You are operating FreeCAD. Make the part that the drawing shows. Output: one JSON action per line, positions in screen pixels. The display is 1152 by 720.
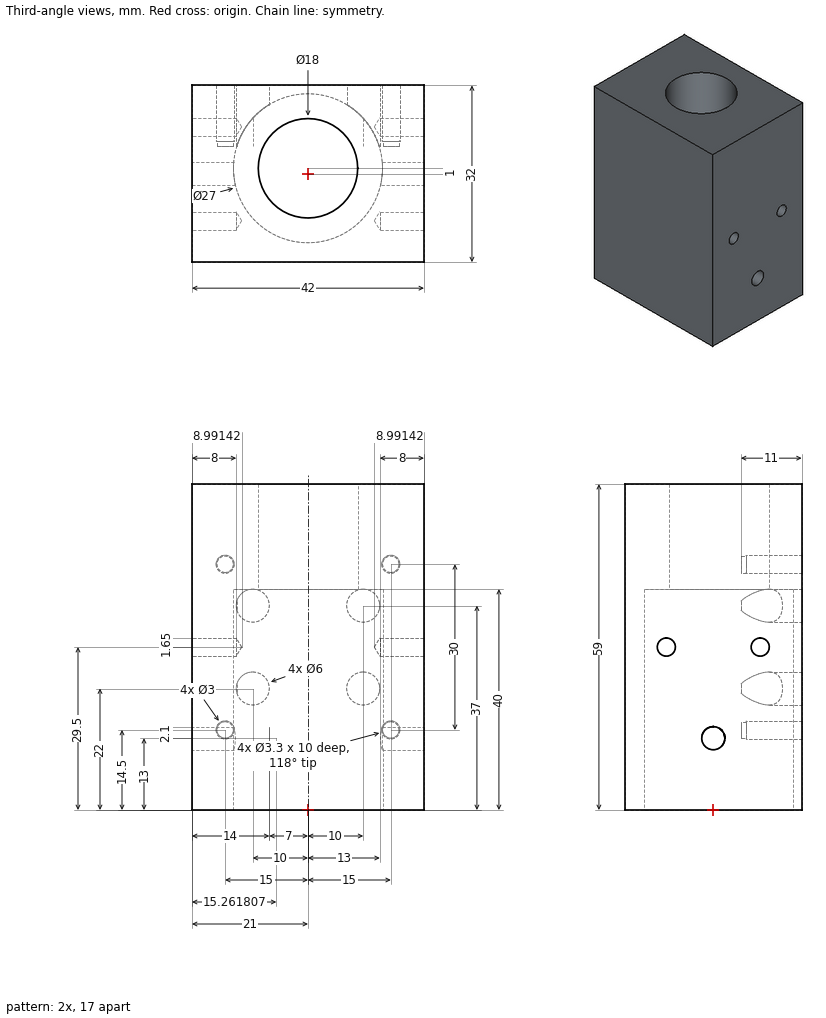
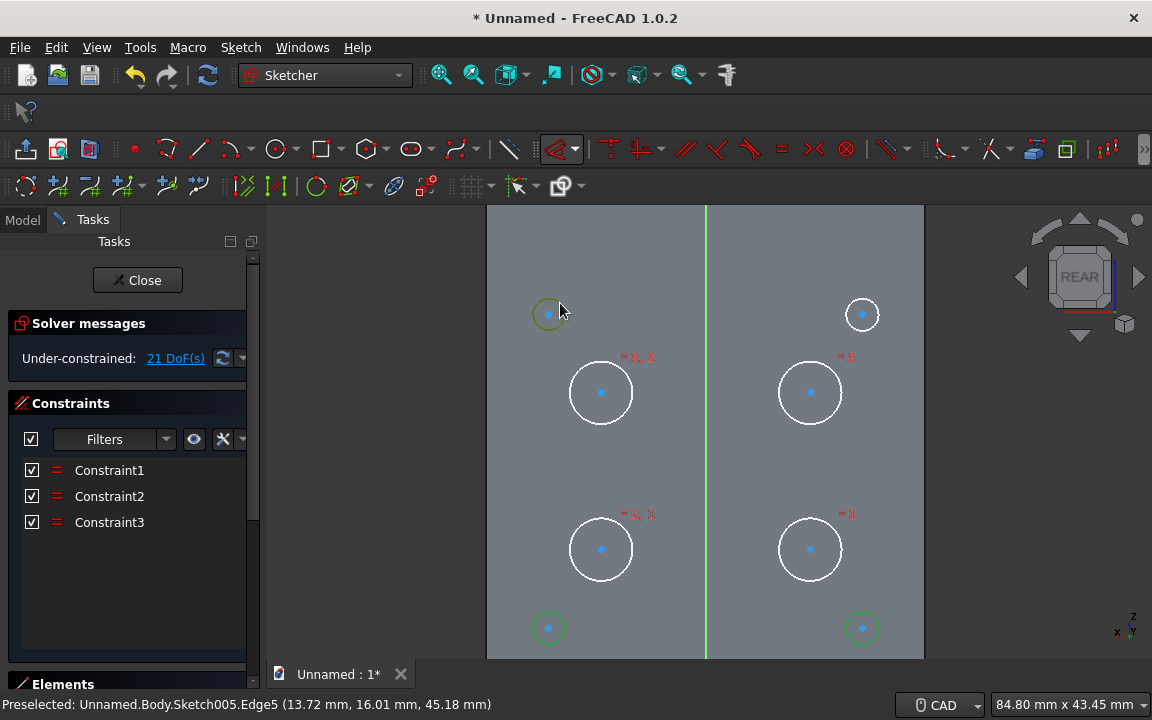
{"action": "left_click", "coordinate": [874, 303]}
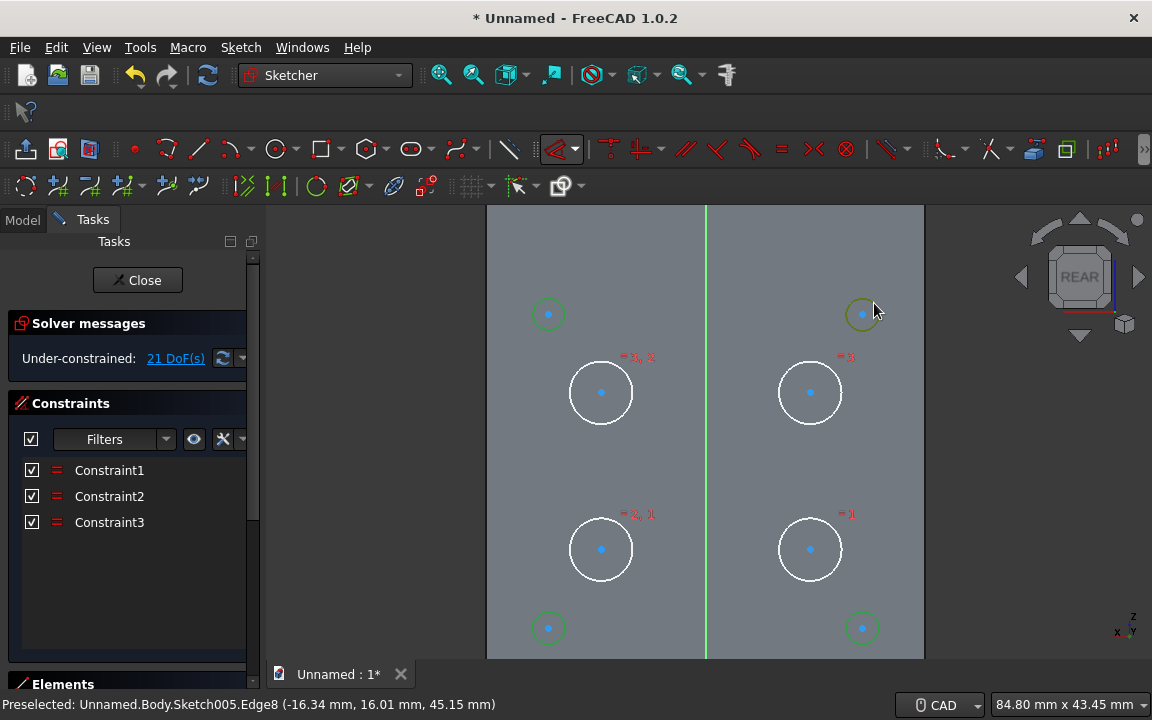
{"action": "left_click", "coordinate": [782, 150]}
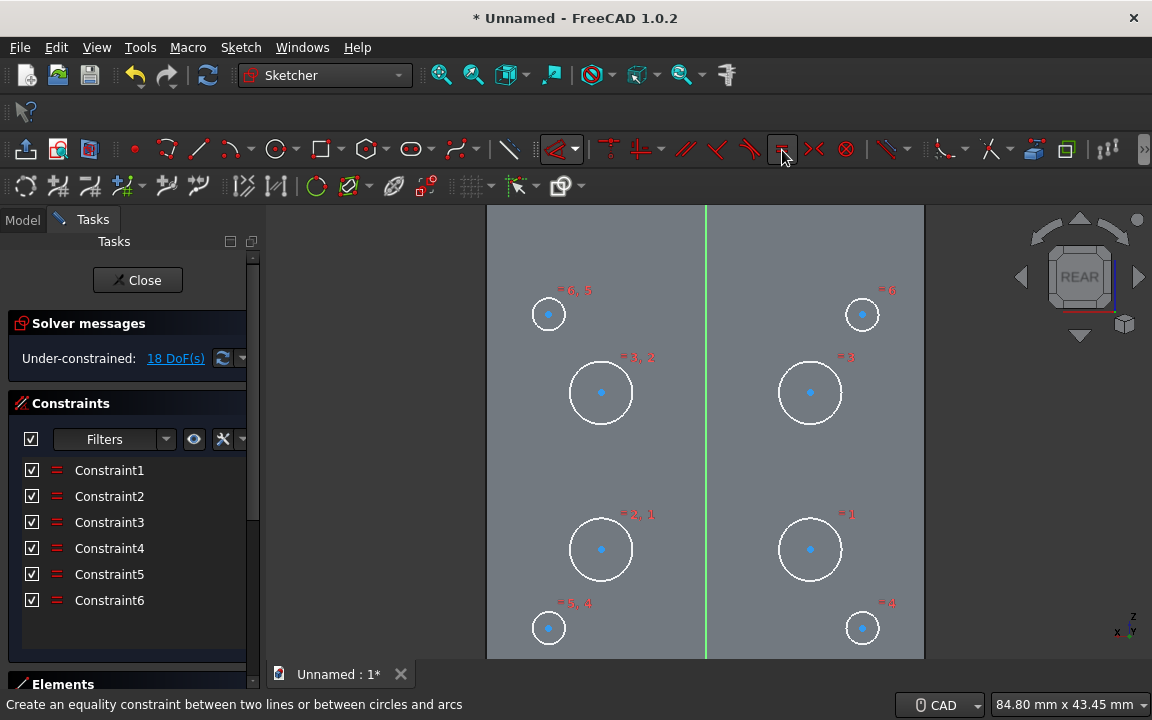
{"action": "left_click", "coordinate": [810, 550]}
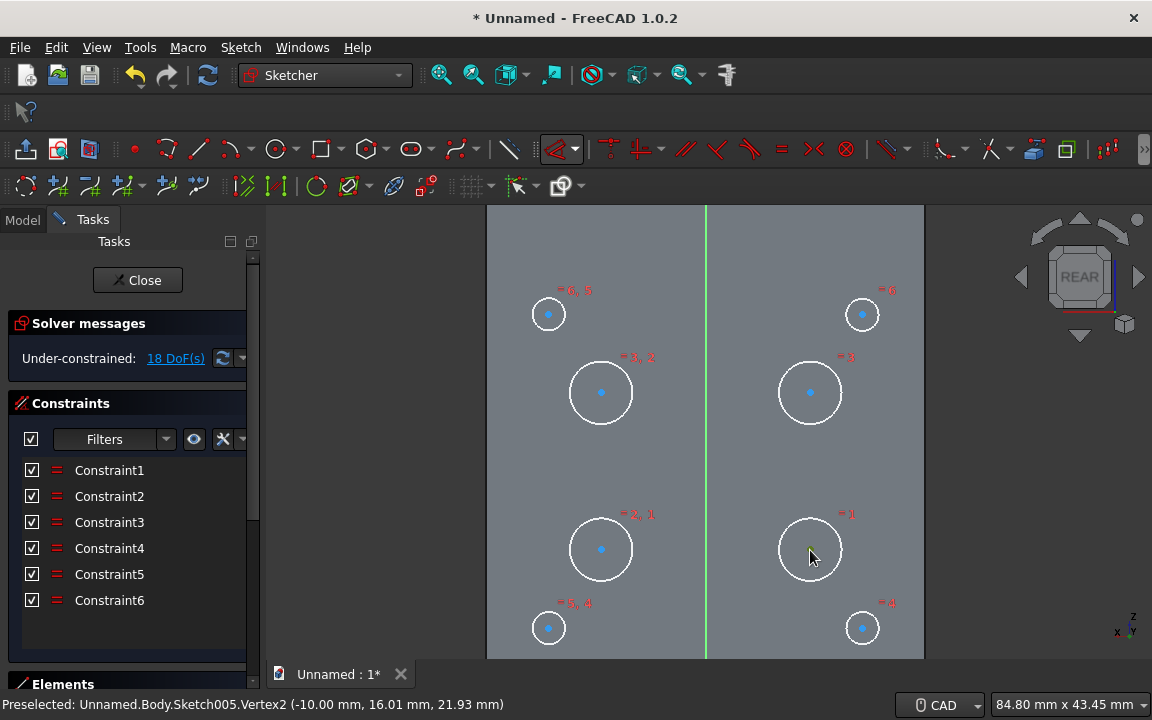
{"action": "left_click", "coordinate": [601, 550]}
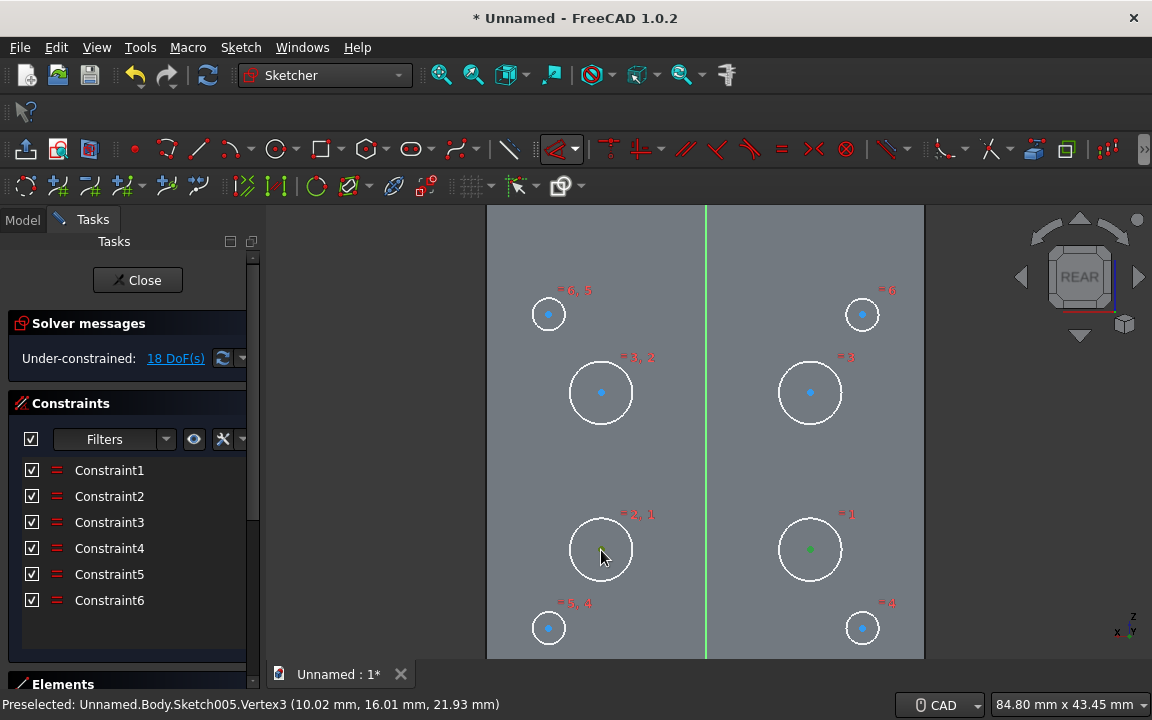
{"action": "left_click", "coordinate": [706, 603]}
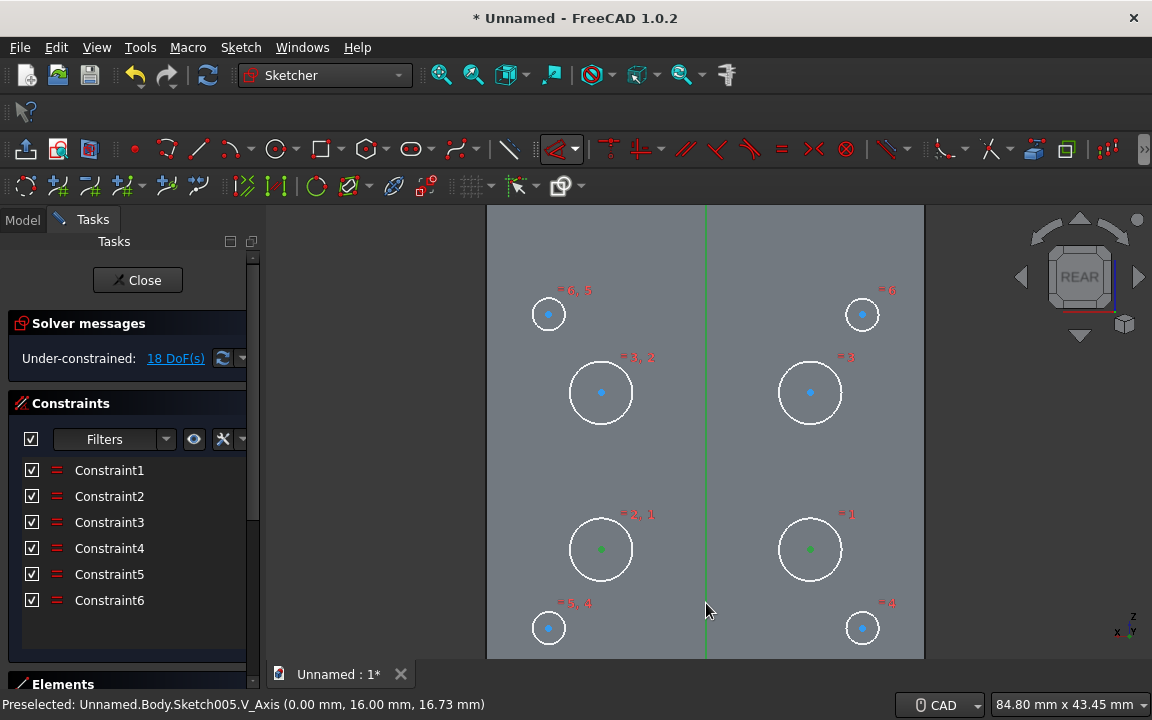
{"action": "key", "text": "s"}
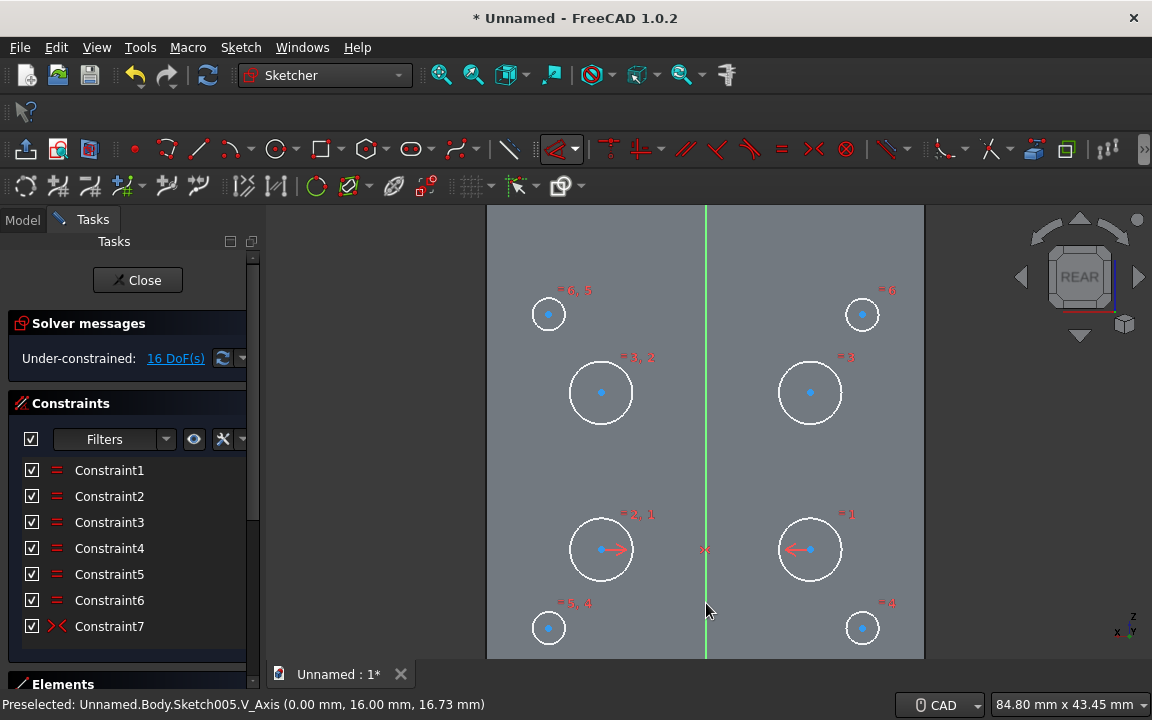
{"action": "left_click", "coordinate": [863, 628]}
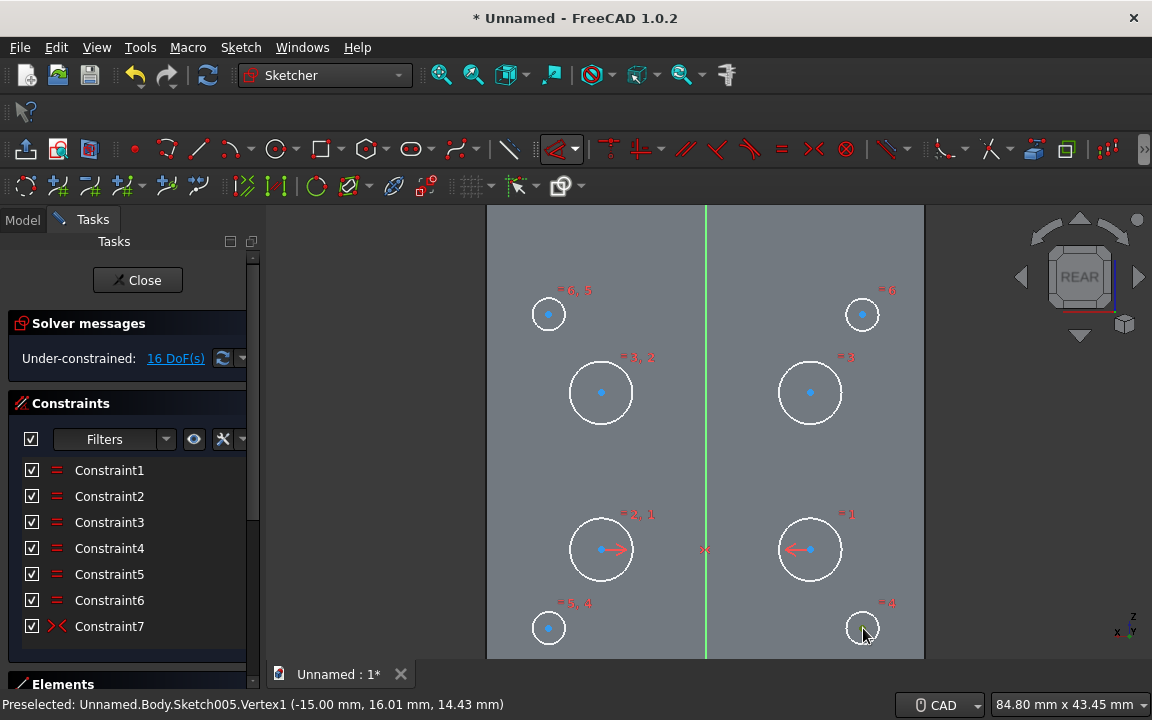
{"action": "left_click", "coordinate": [549, 628]}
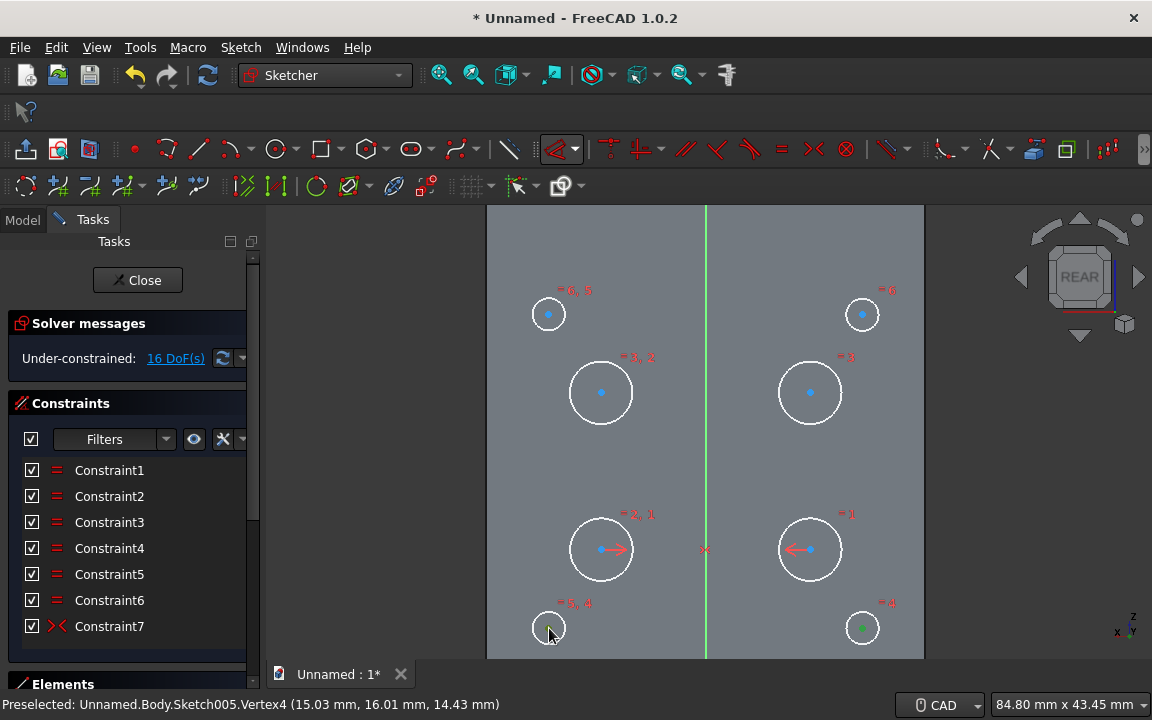
{"action": "left_click", "coordinate": [706, 603]}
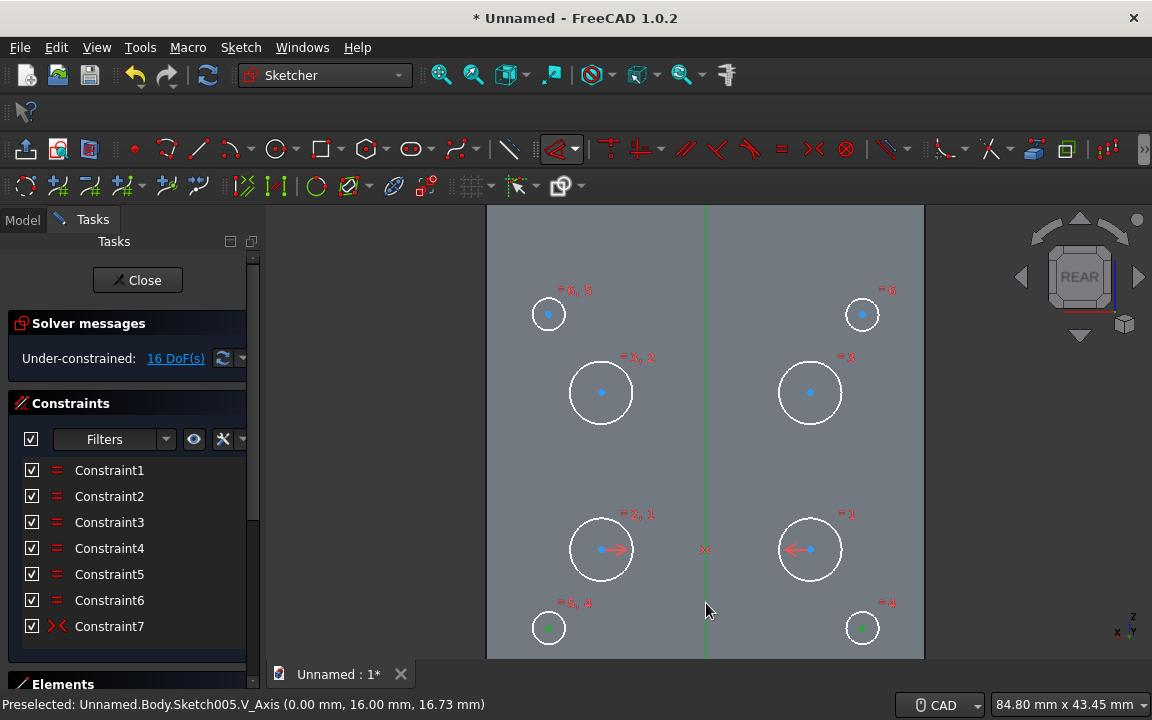
{"action": "left_click", "coordinate": [814, 150]}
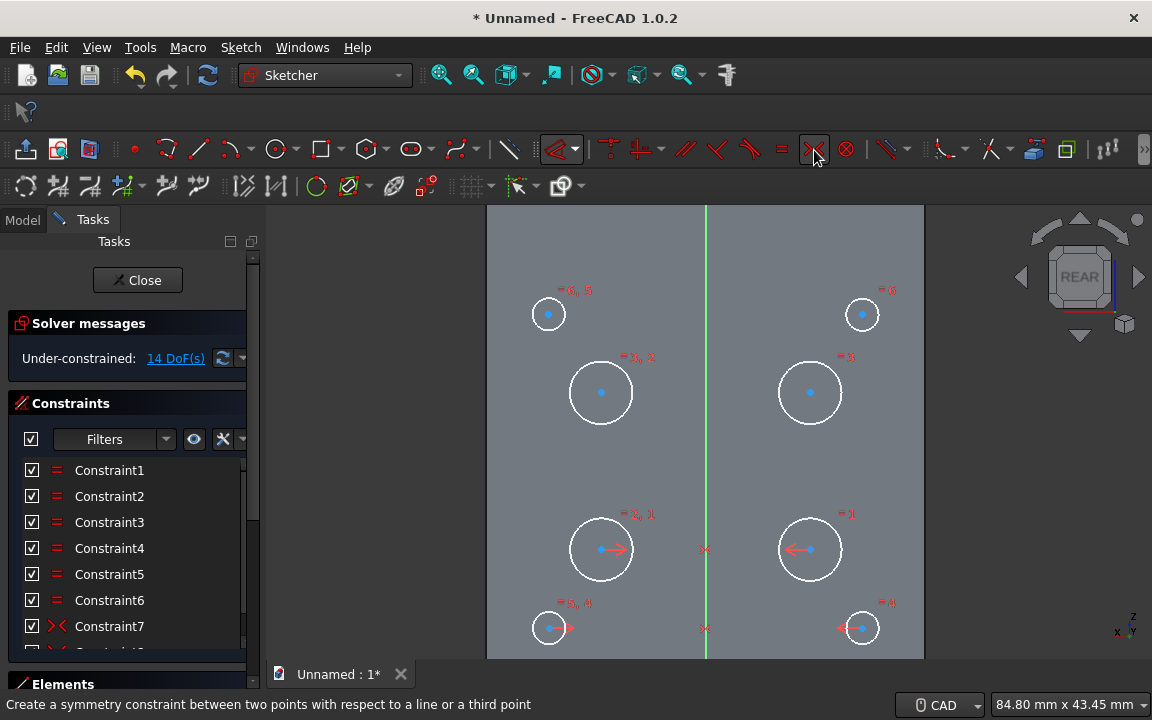
{"action": "left_click", "coordinate": [601, 393]}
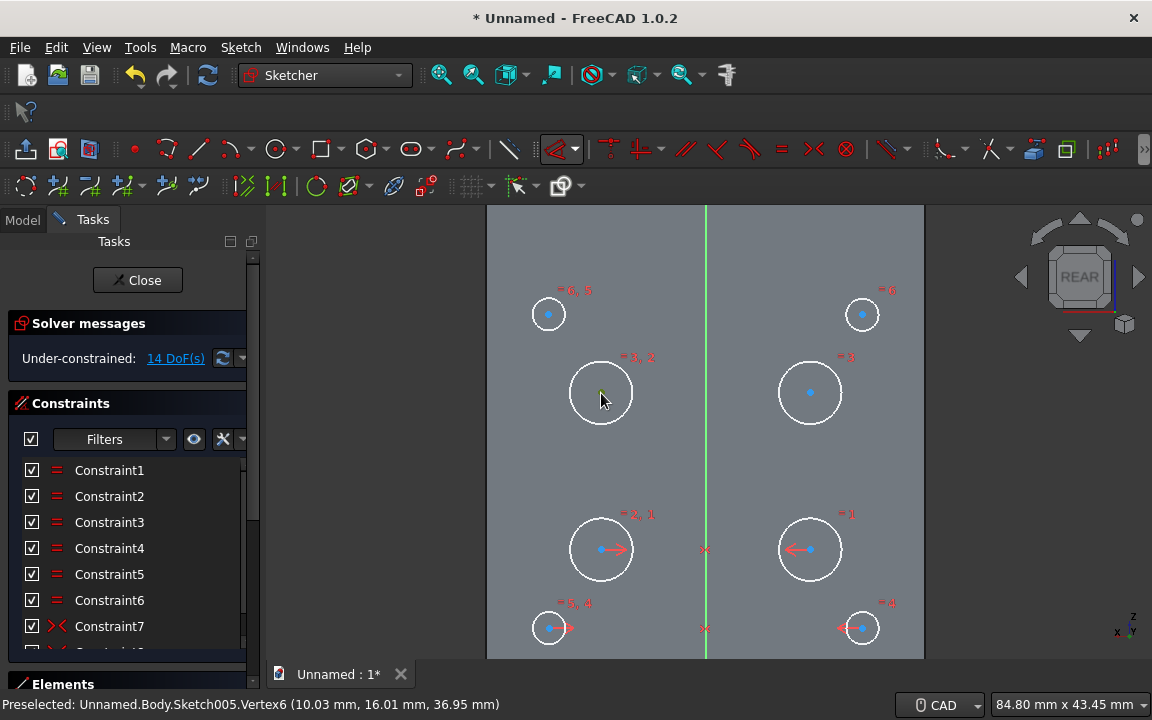
{"action": "left_click", "coordinate": [810, 393]}